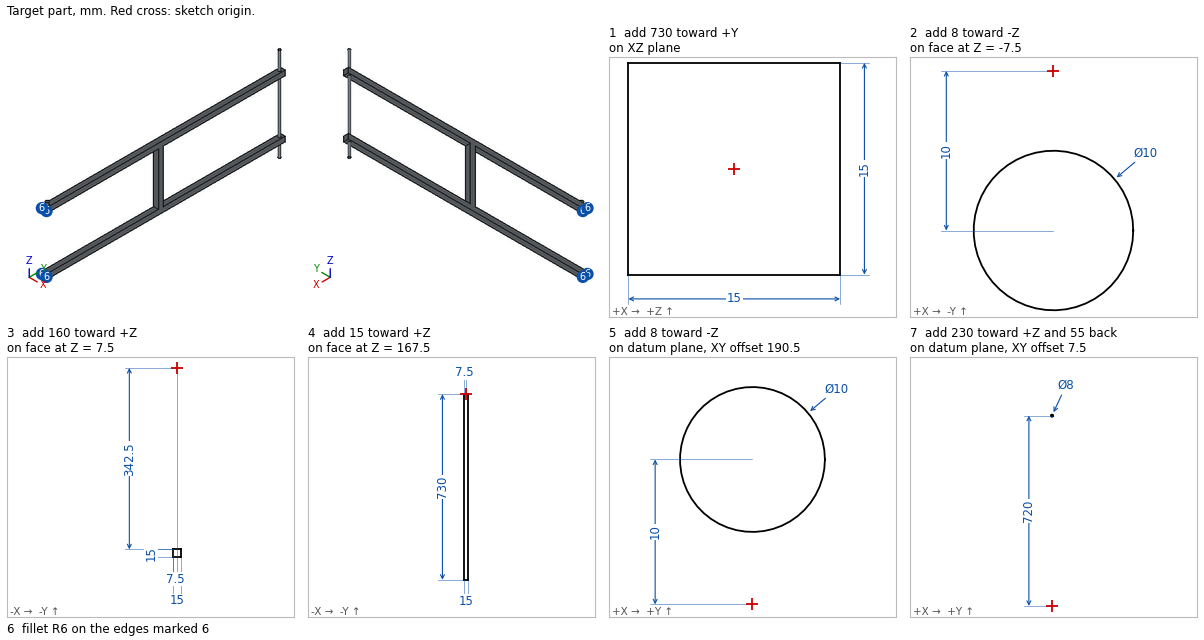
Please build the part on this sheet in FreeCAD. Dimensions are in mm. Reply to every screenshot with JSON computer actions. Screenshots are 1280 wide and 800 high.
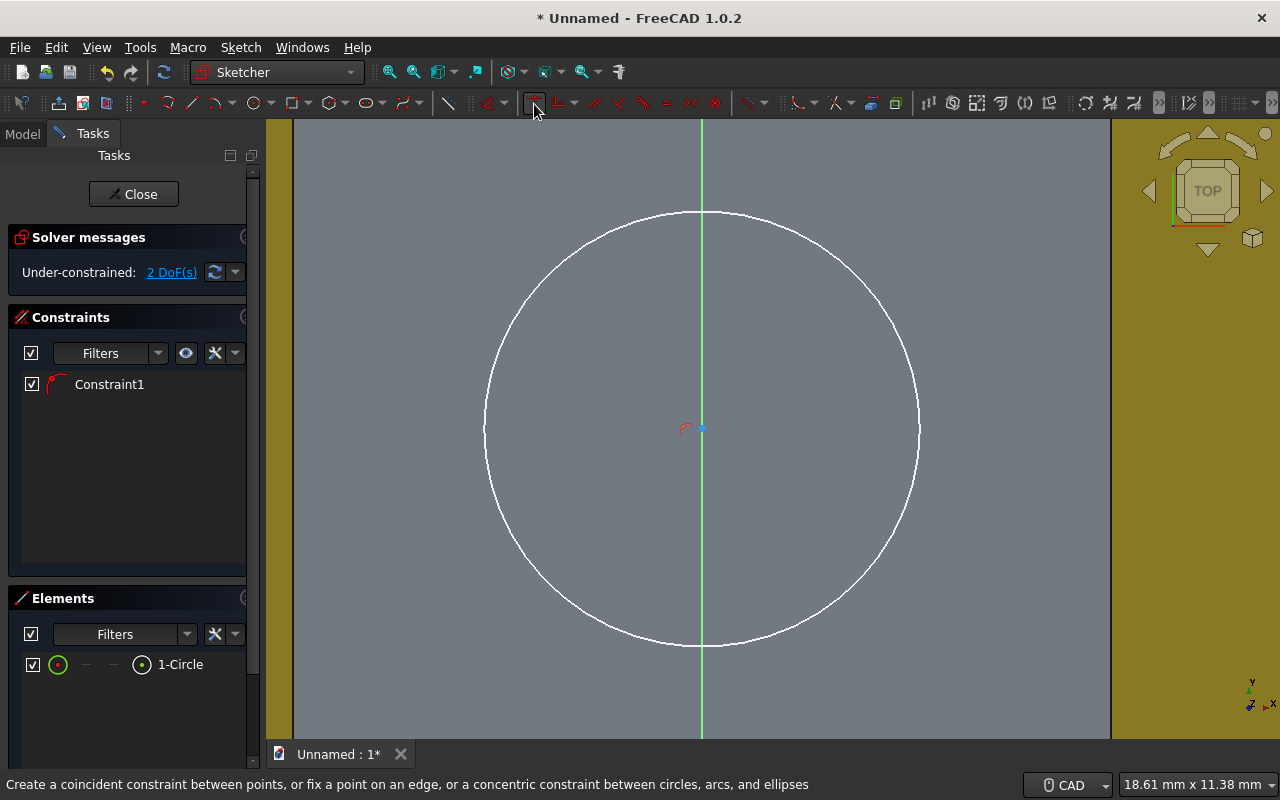
{"action": "left_click", "coordinate": [488, 104]}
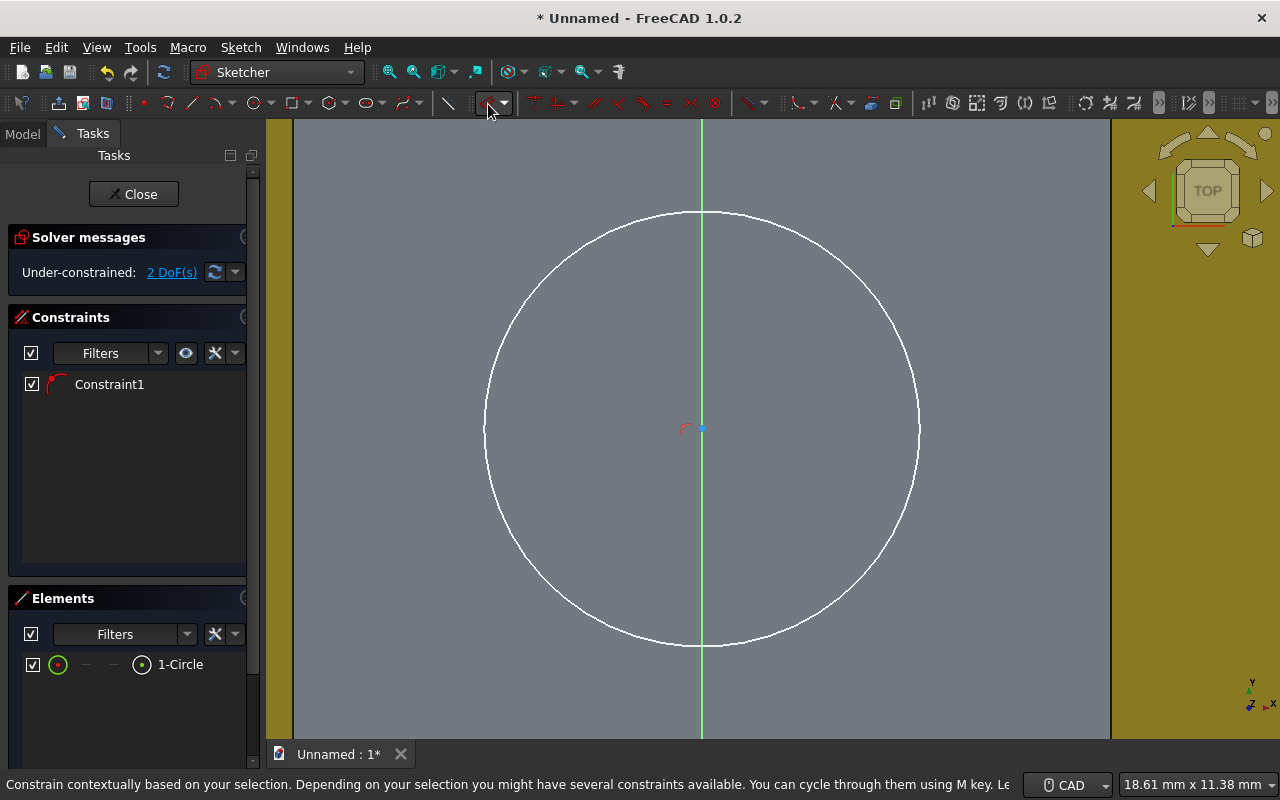
{"action": "left_click", "coordinate": [856, 275]}
{"action": "left_click", "coordinate": [879, 252]}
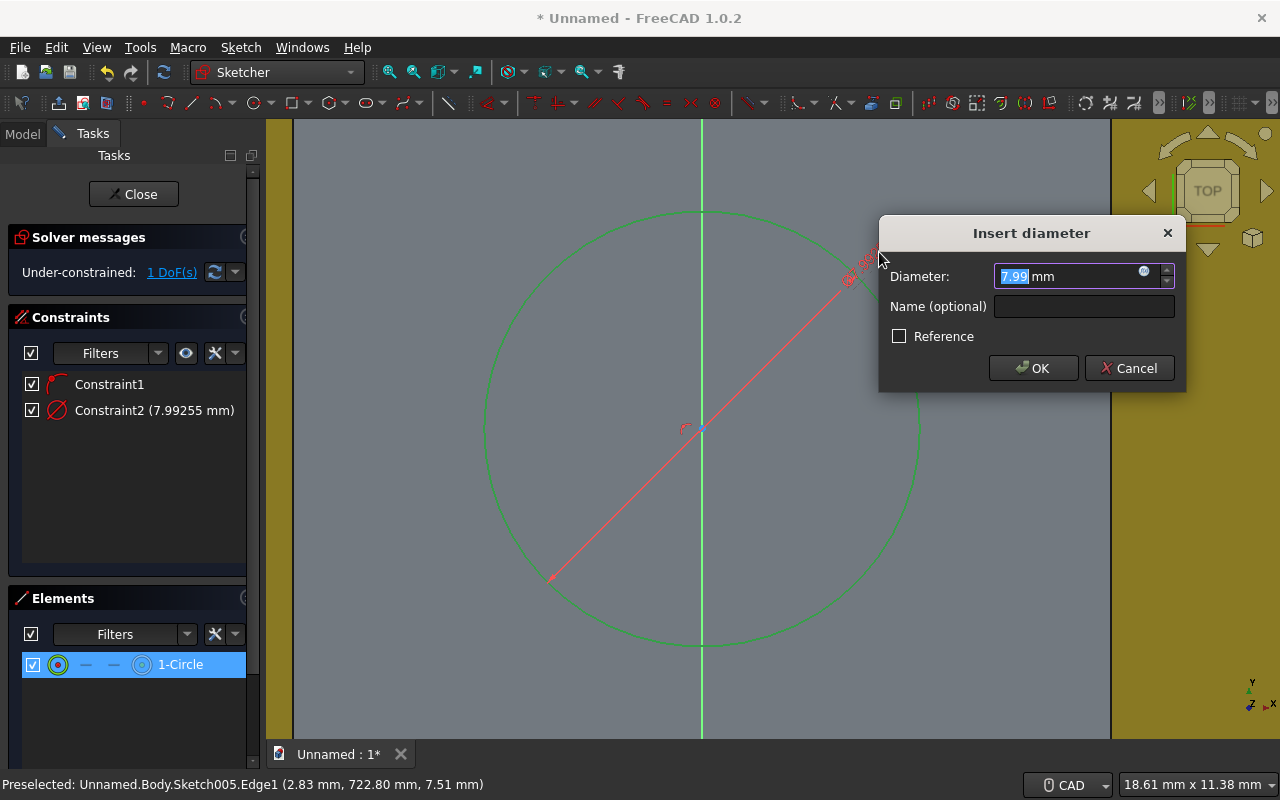
{"action": "type", "text": "8"}
{"action": "key", "text": "Return"}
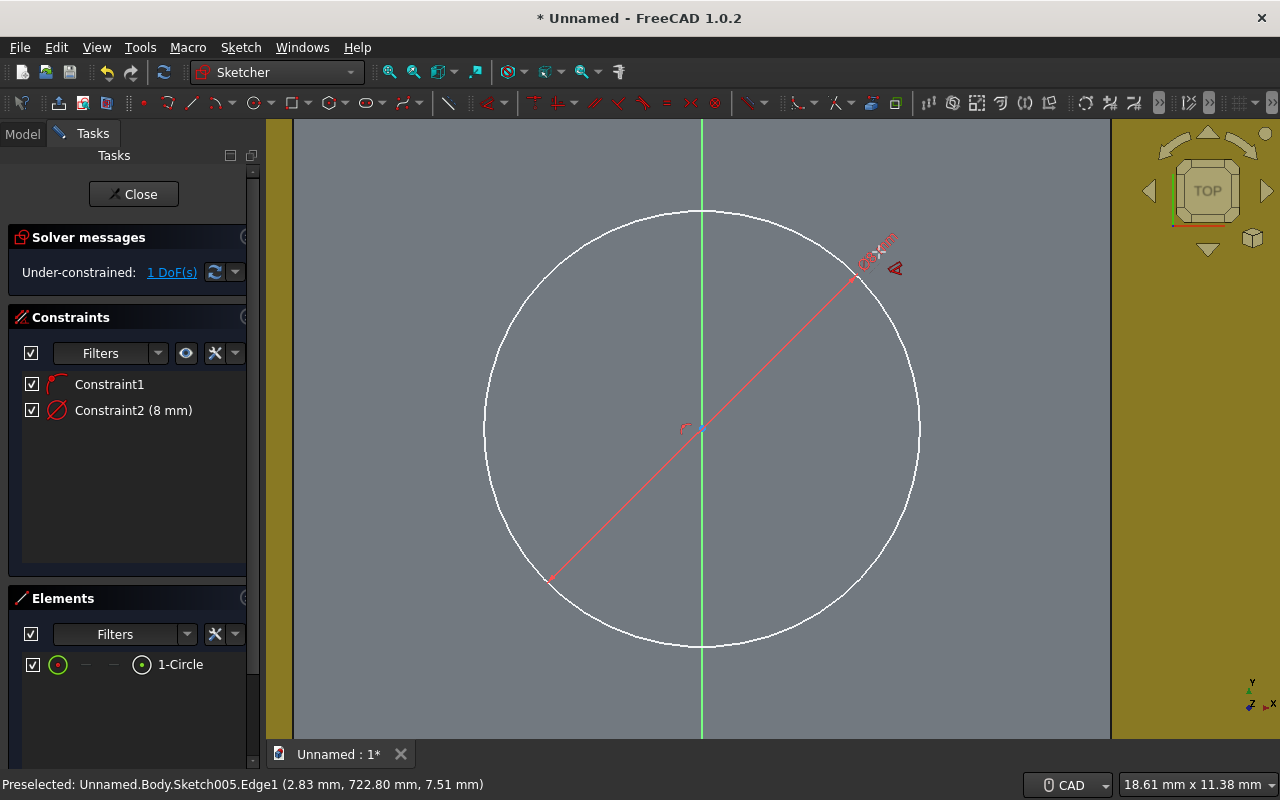
{"action": "left_click", "coordinate": [702, 429]}
{"action": "left_click", "coordinate": [736, 570]}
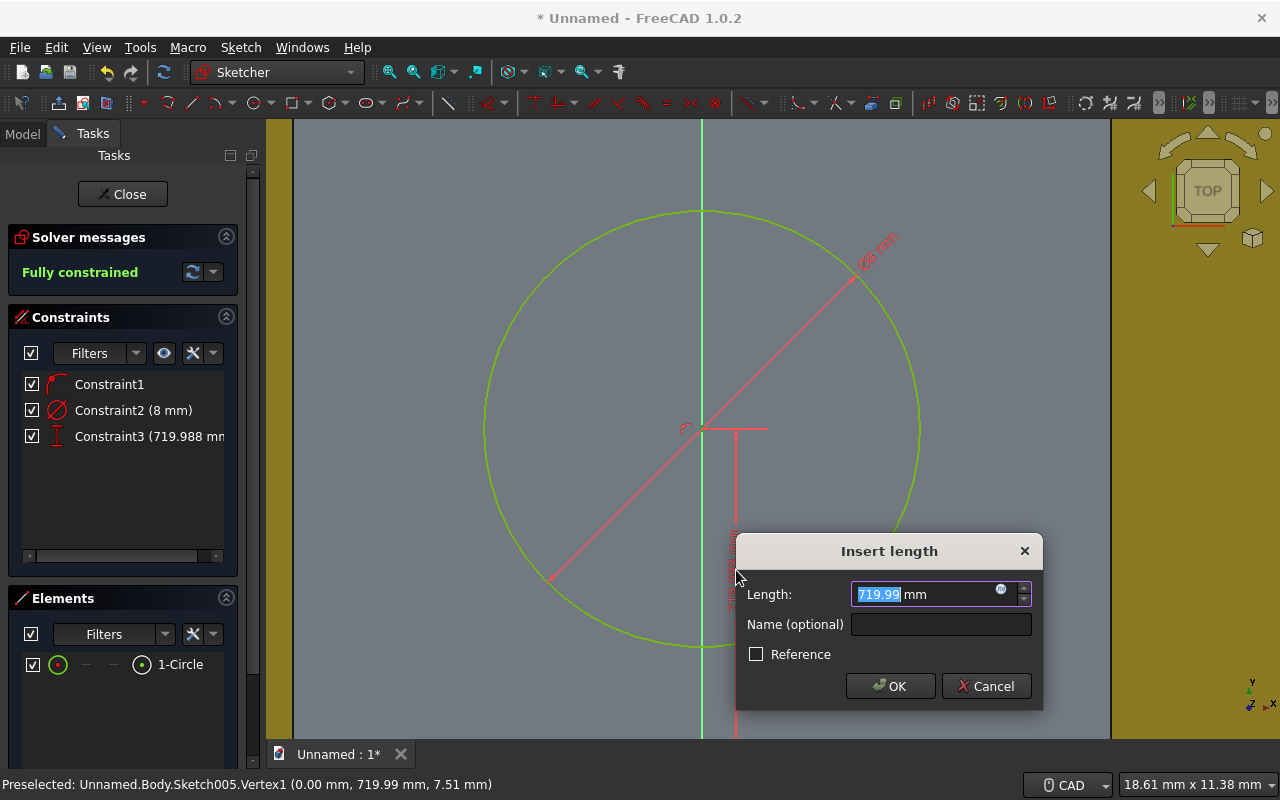
{"action": "type", "text": "720"}
{"action": "key", "text": "Return"}
{"action": "key", "text": "Escape"}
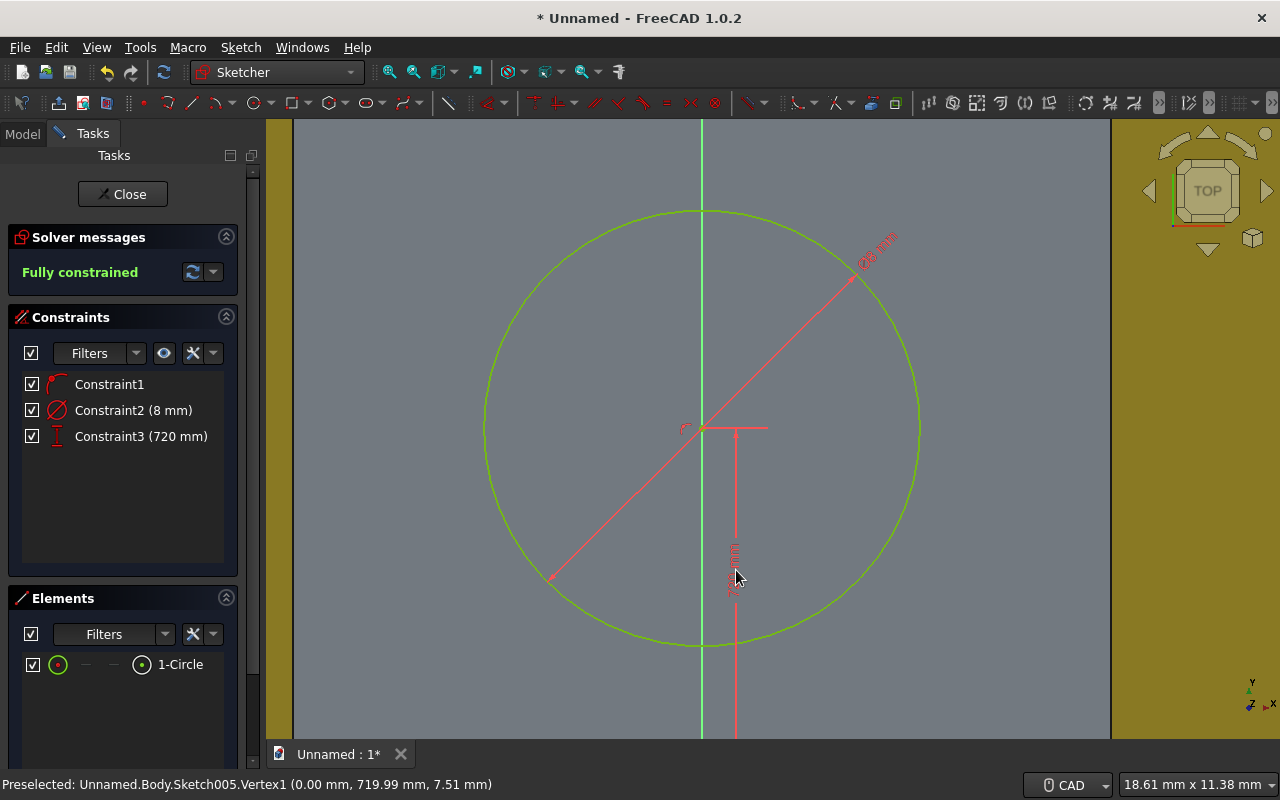
{"action": "left_click", "coordinate": [123, 194]}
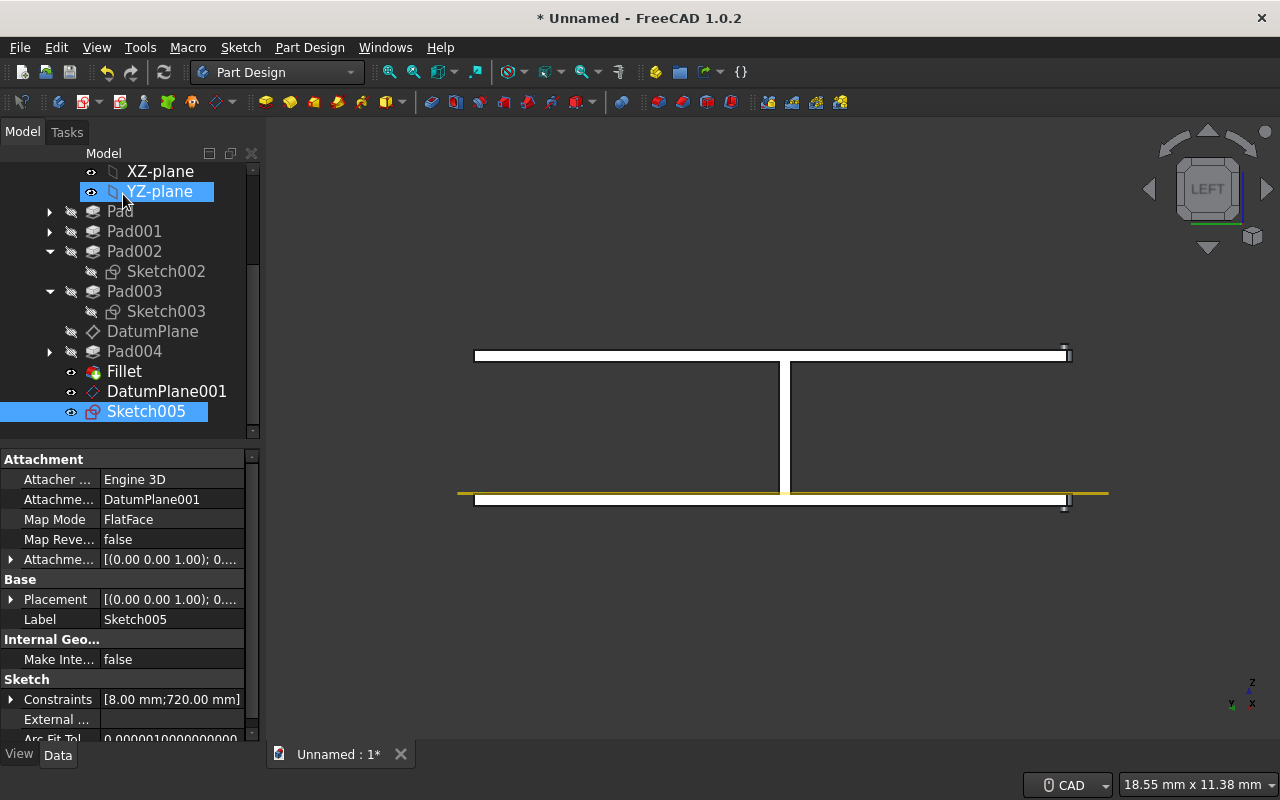
{"action": "left_click", "coordinate": [266, 102]}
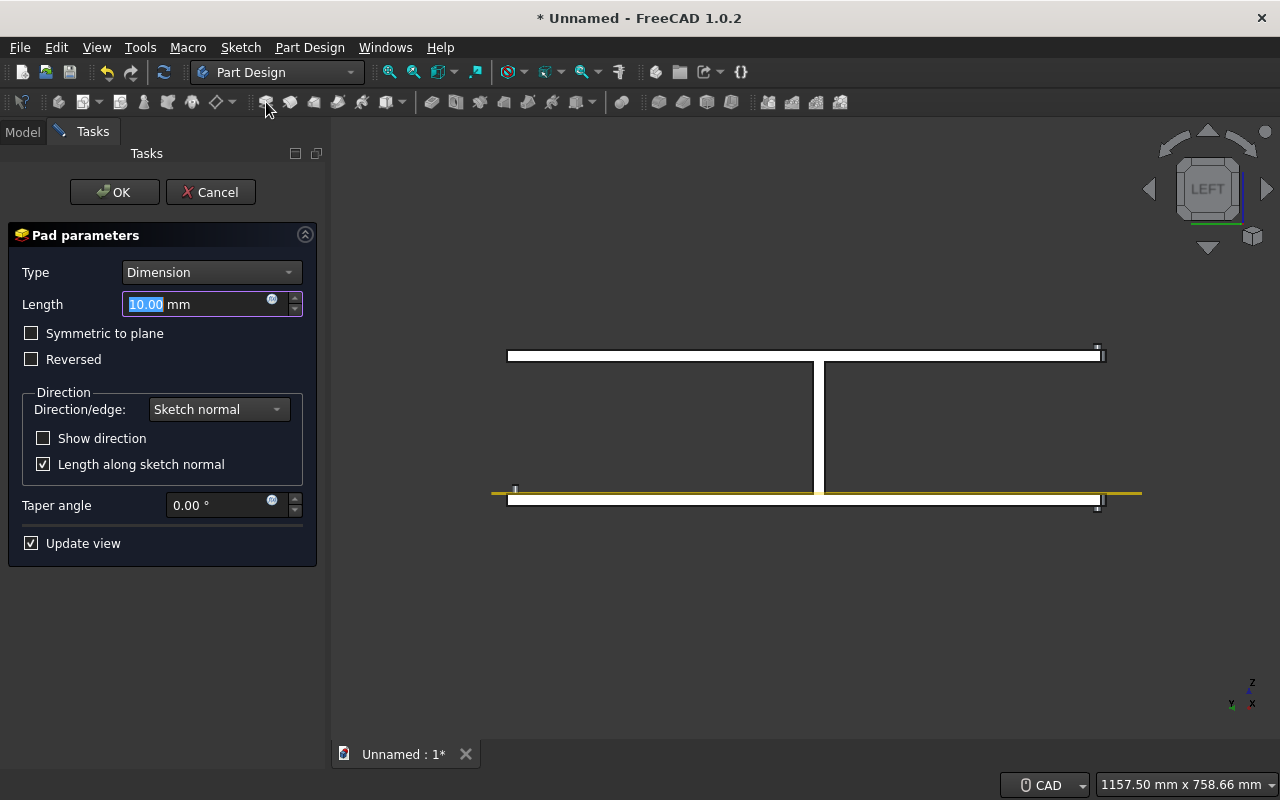
{"action": "left_click", "coordinate": [212, 272]}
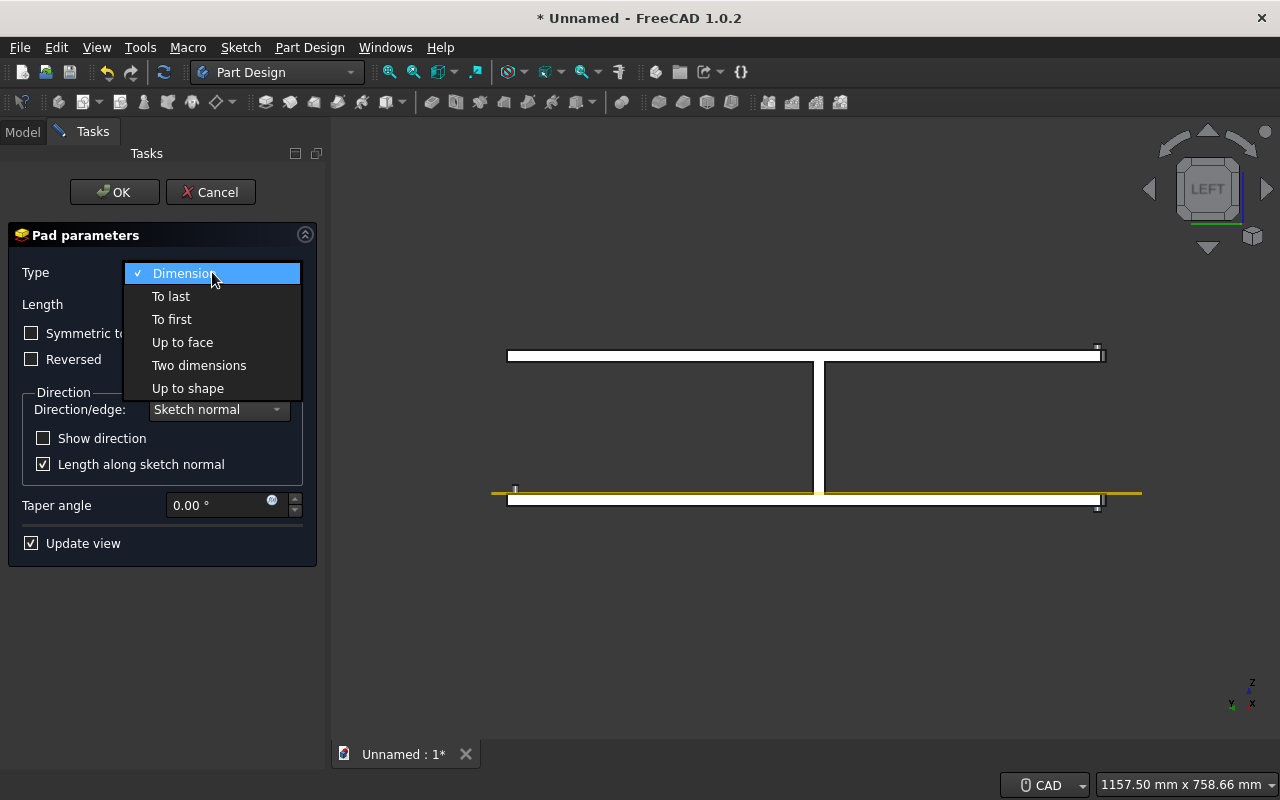
{"action": "left_click", "coordinate": [212, 366]}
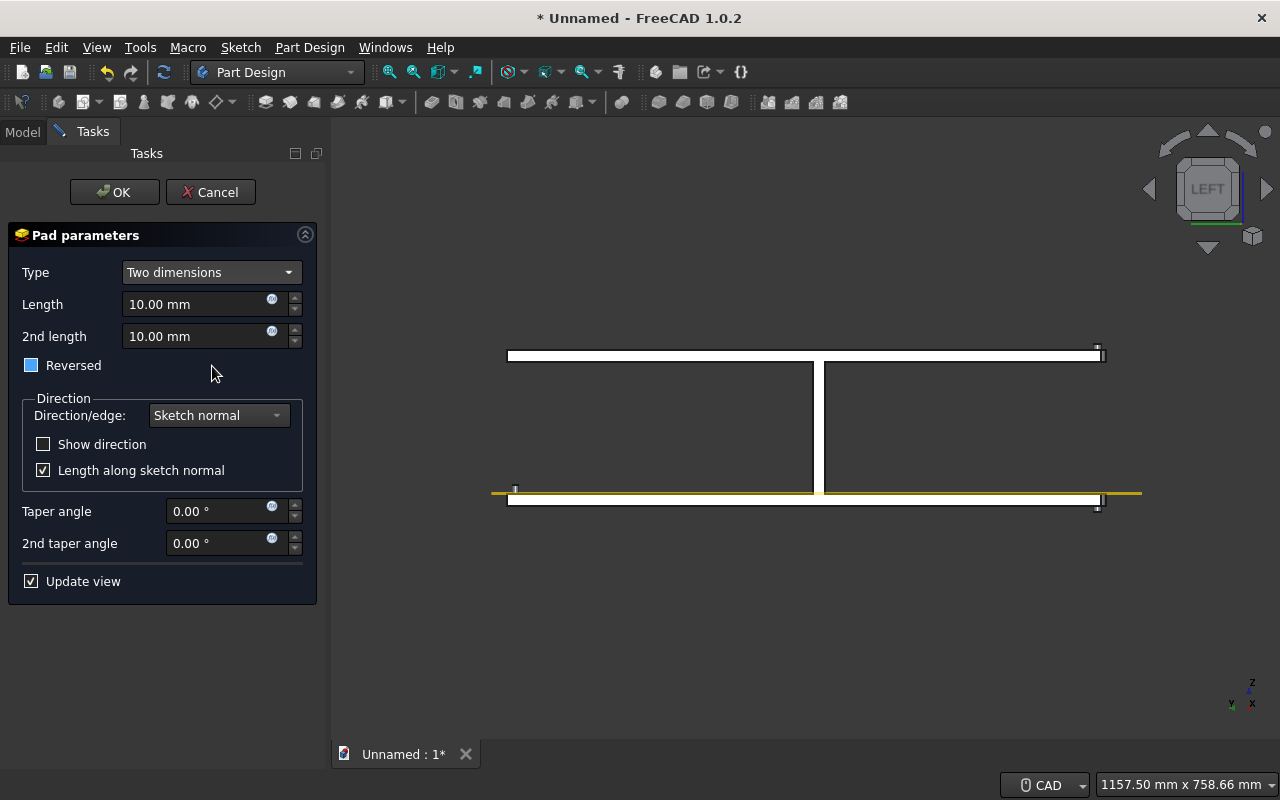
{"action": "triple_click", "coordinate": [204, 304]}